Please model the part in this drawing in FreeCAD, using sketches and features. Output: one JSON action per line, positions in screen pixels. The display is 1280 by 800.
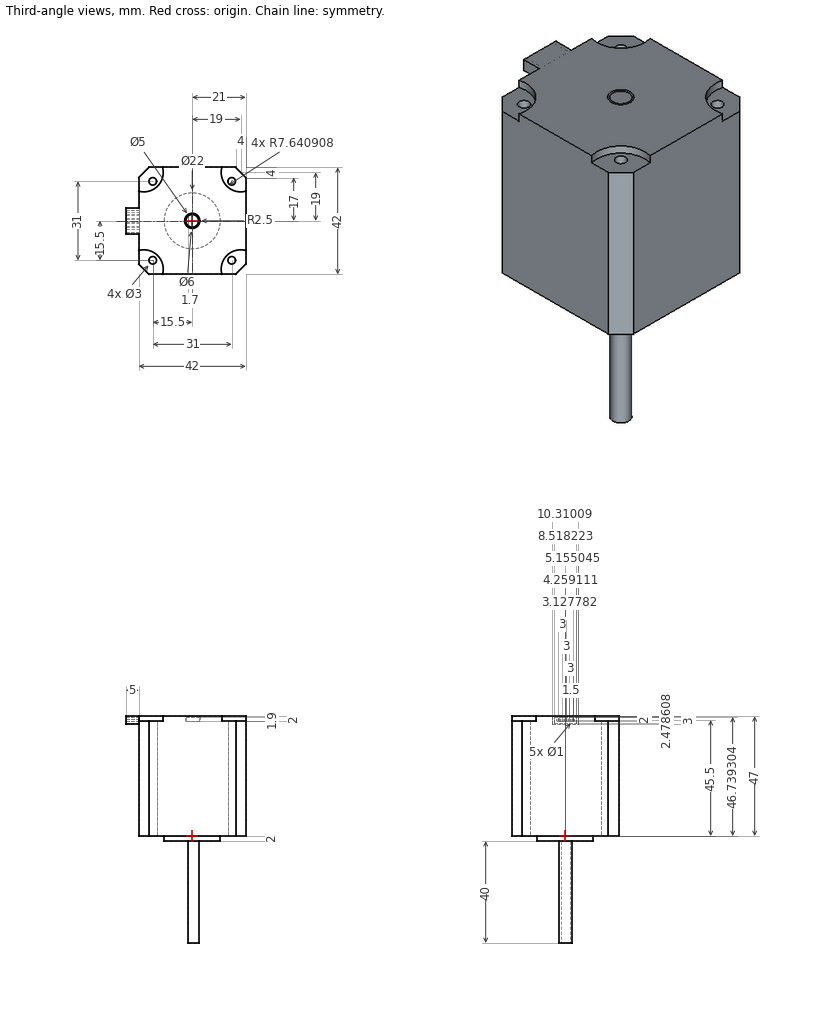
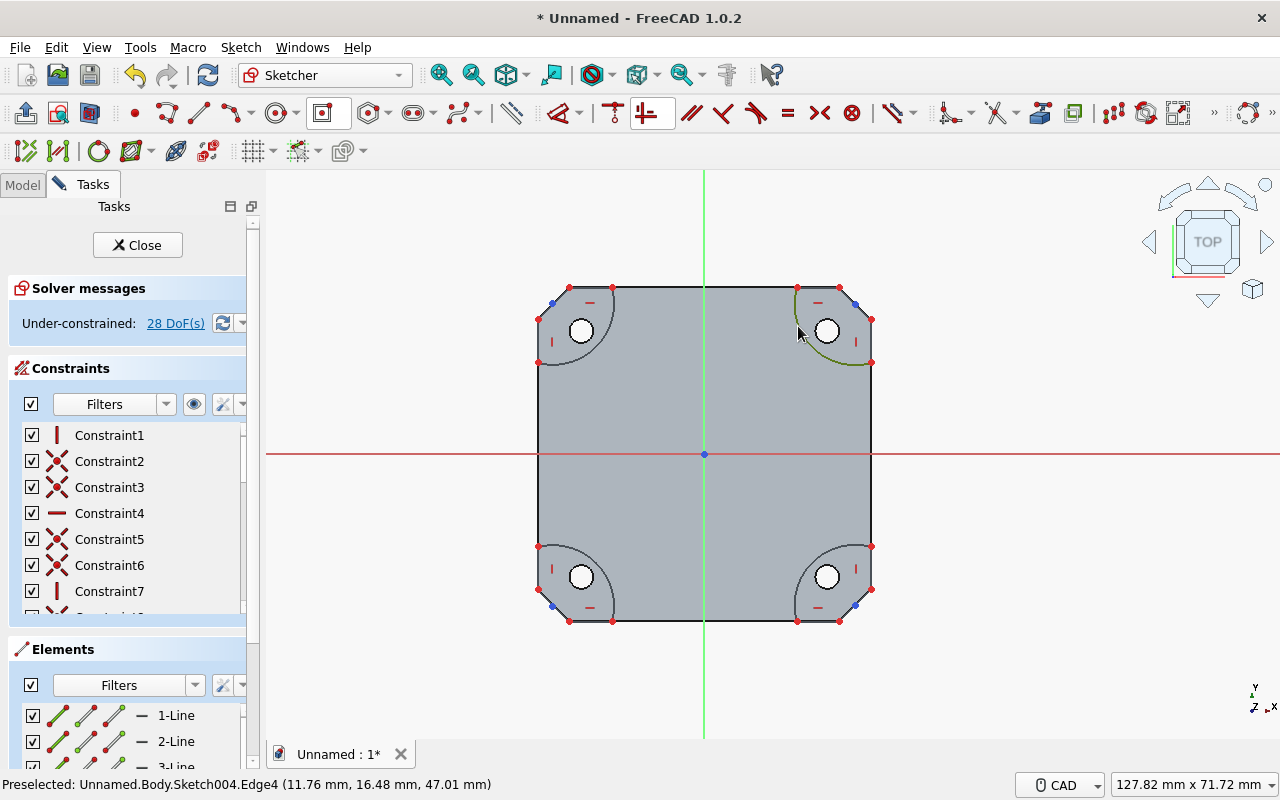
{"action": "left_click", "coordinate": [610, 585]}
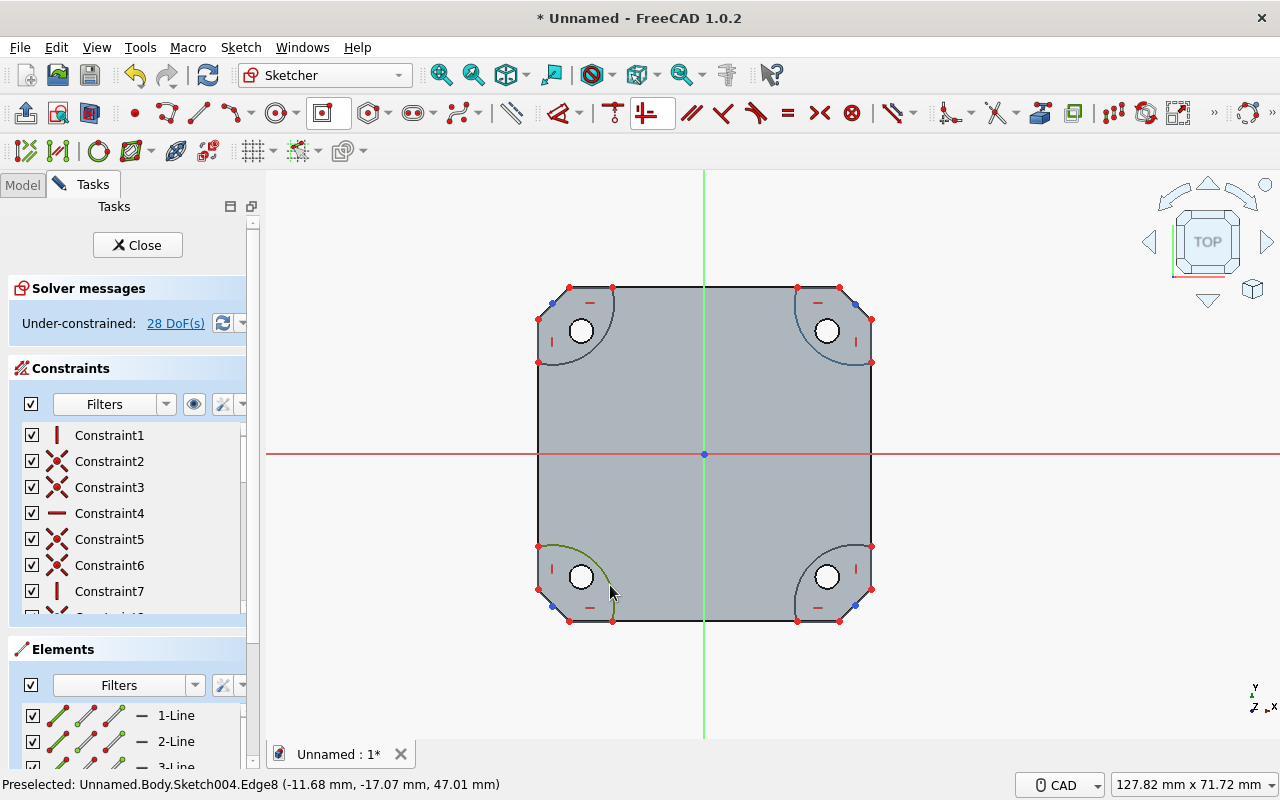
{"action": "left_click", "coordinate": [575, 361]}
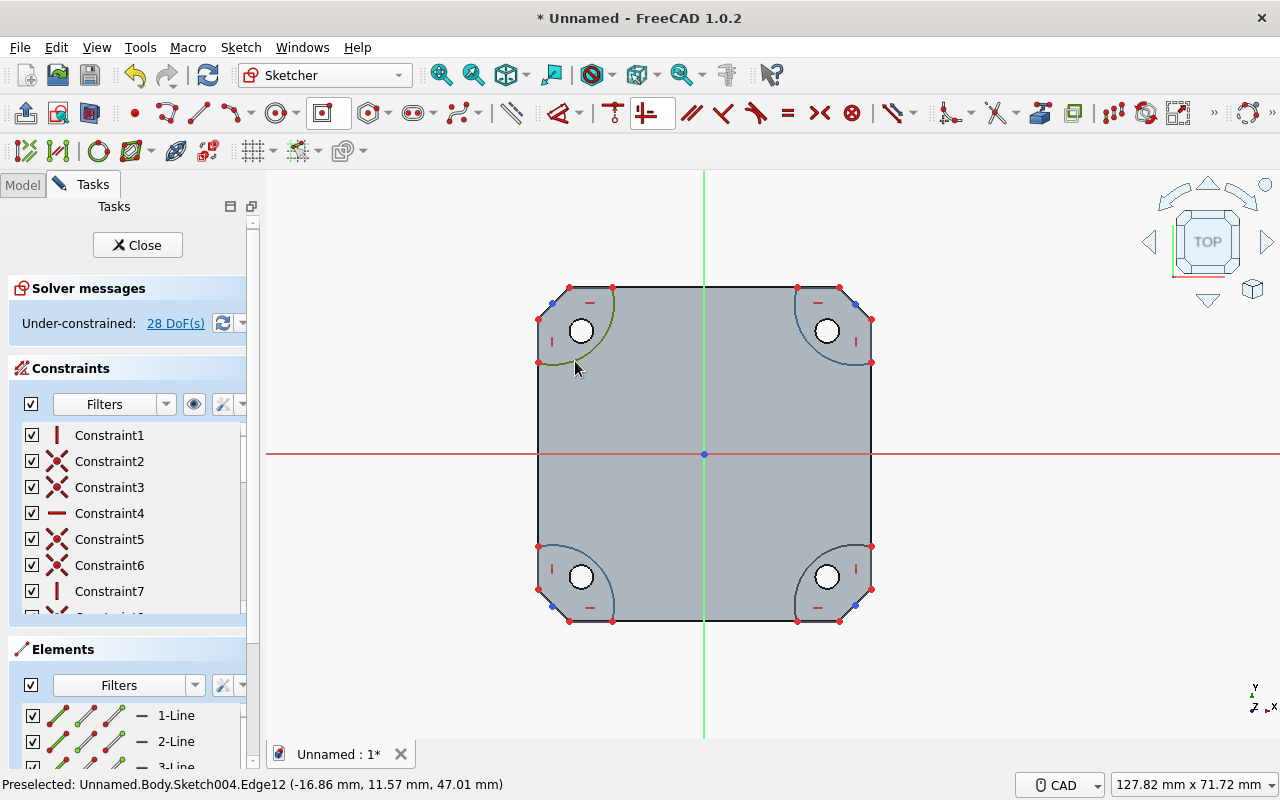
{"action": "left_click", "coordinate": [833, 549]}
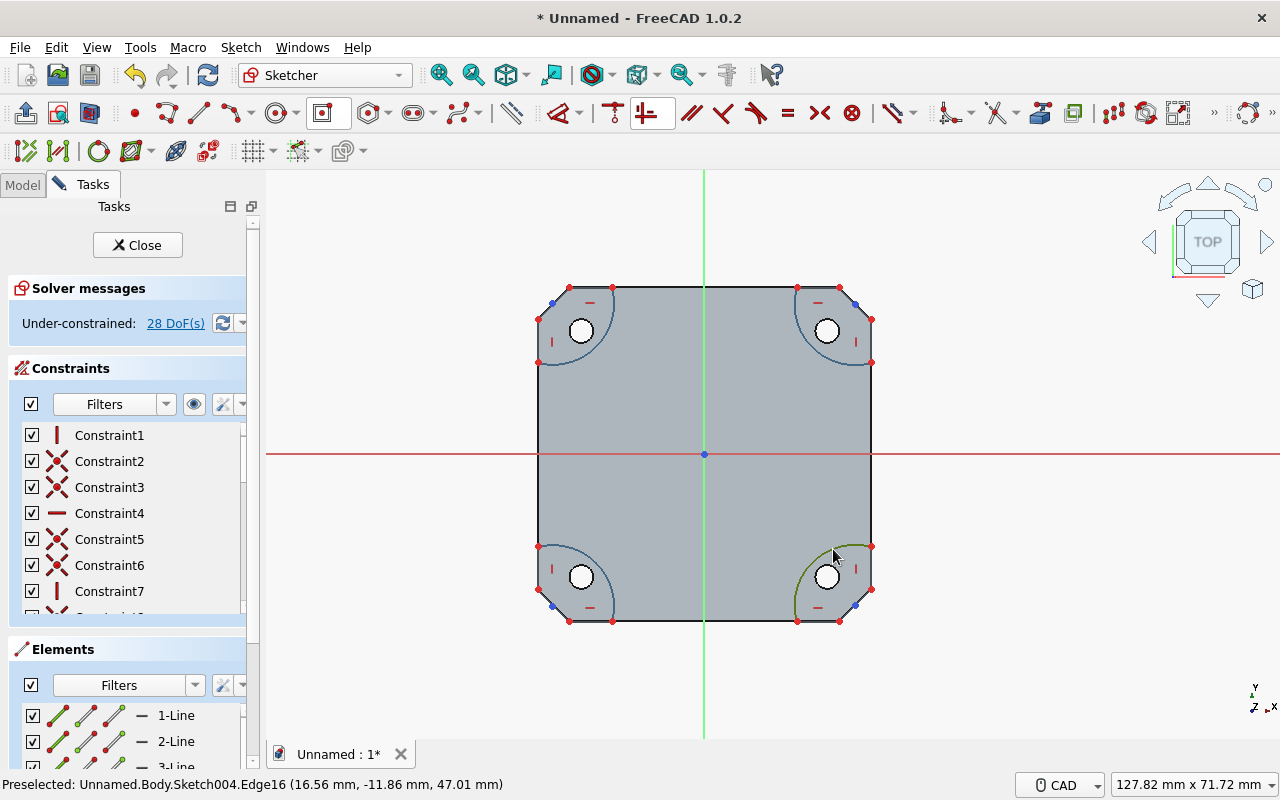
{"action": "key", "text": "e"}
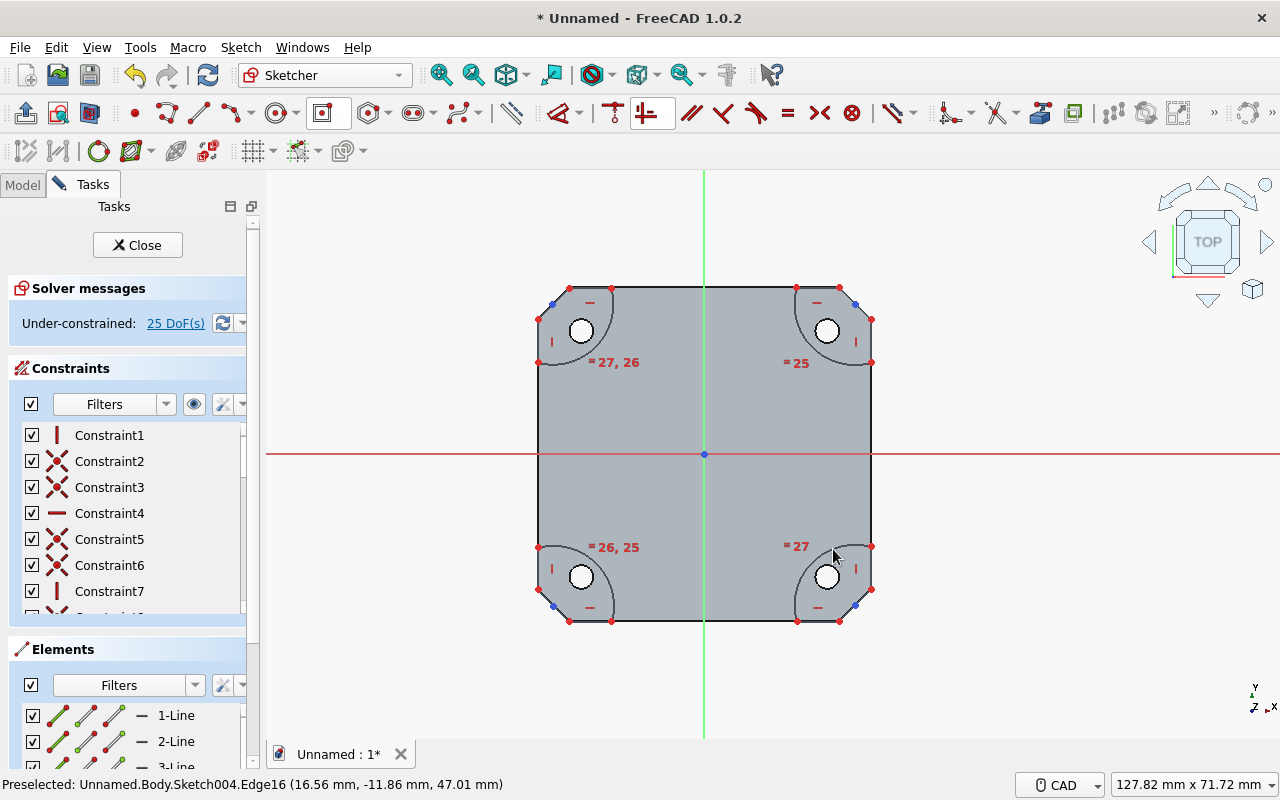
{"action": "left_click", "coordinate": [855, 305]}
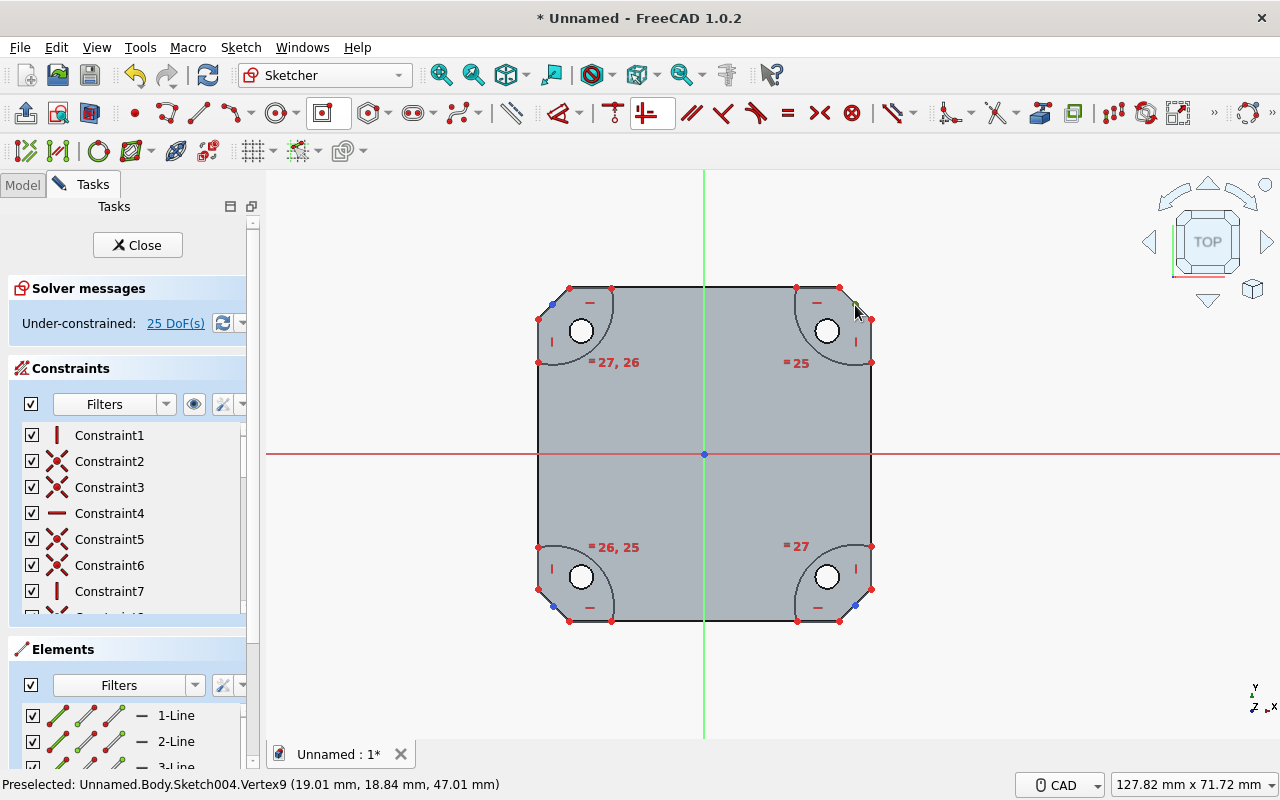
{"action": "left_click", "coordinate": [553, 304]}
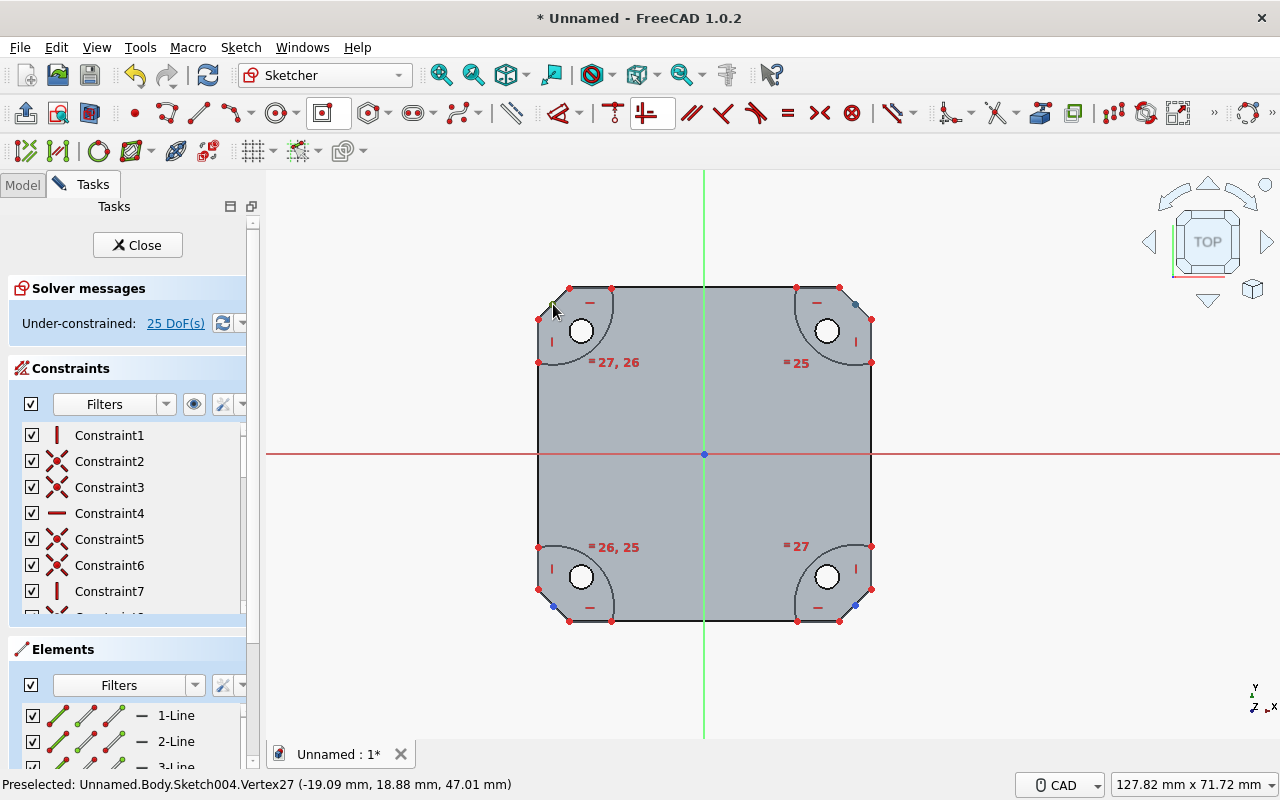
{"action": "left_click", "coordinate": [704, 674]}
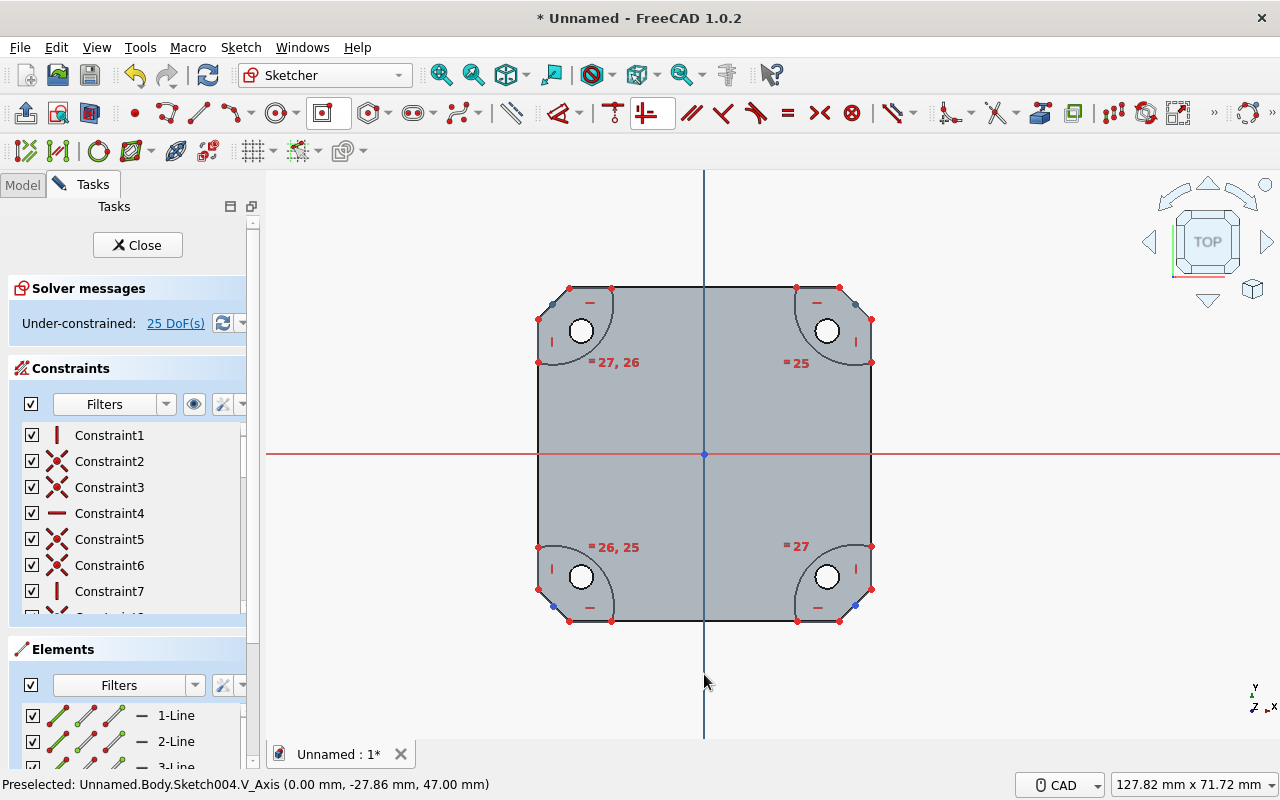
{"action": "key", "text": "s"}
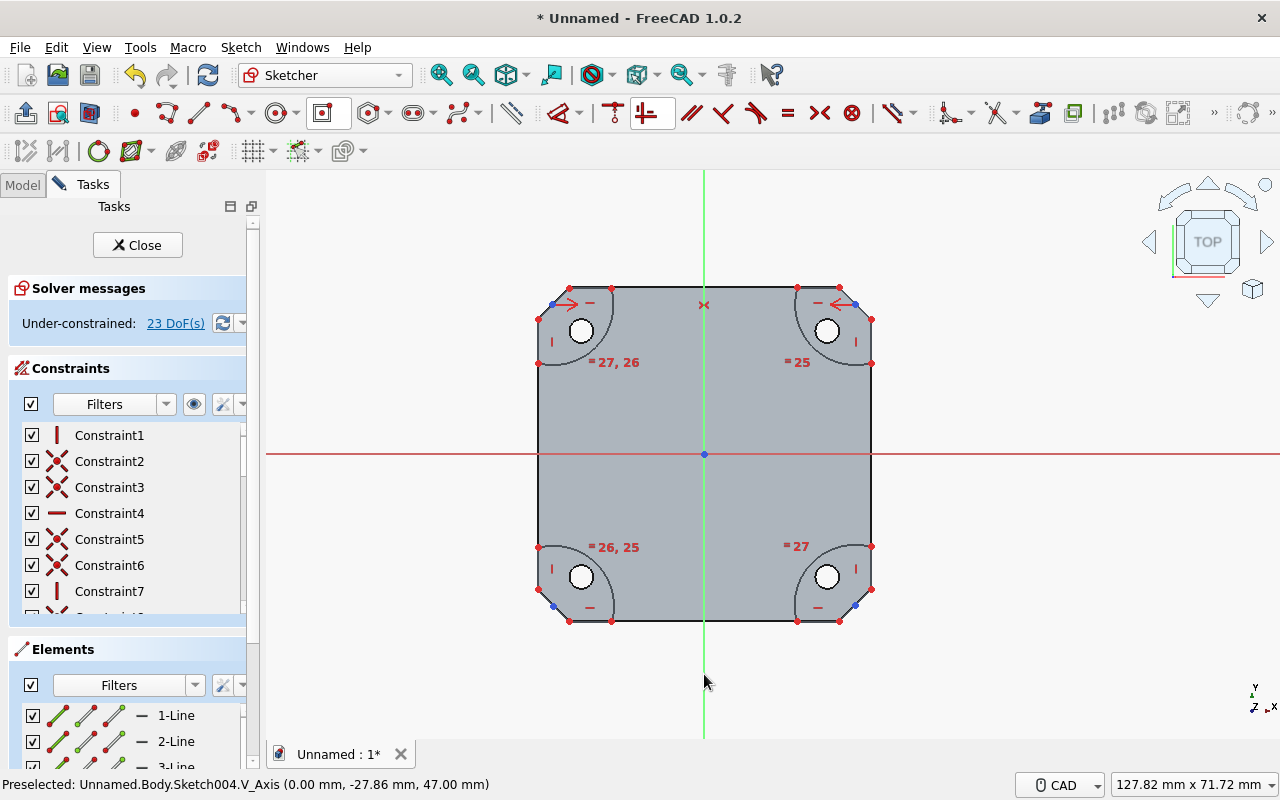
{"action": "left_click", "coordinate": [553, 606]}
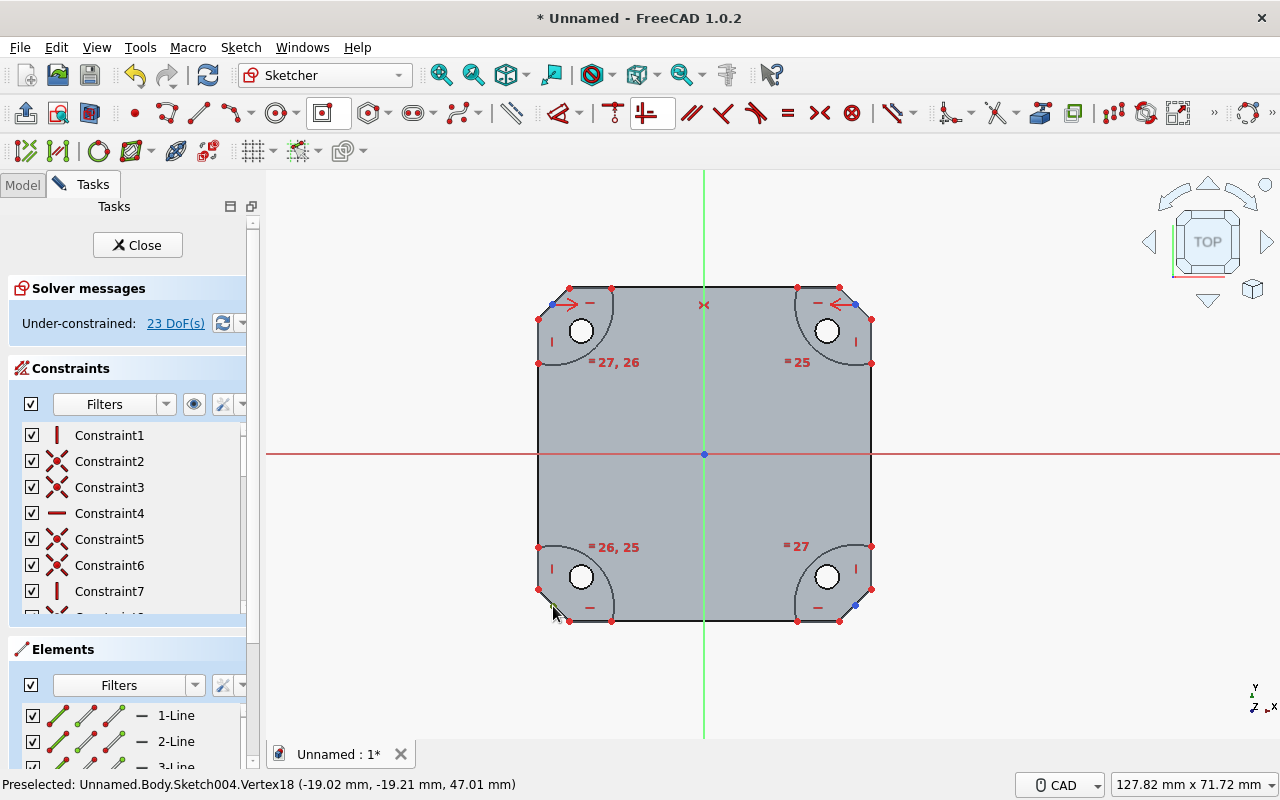
{"action": "left_click", "coordinate": [553, 305]}